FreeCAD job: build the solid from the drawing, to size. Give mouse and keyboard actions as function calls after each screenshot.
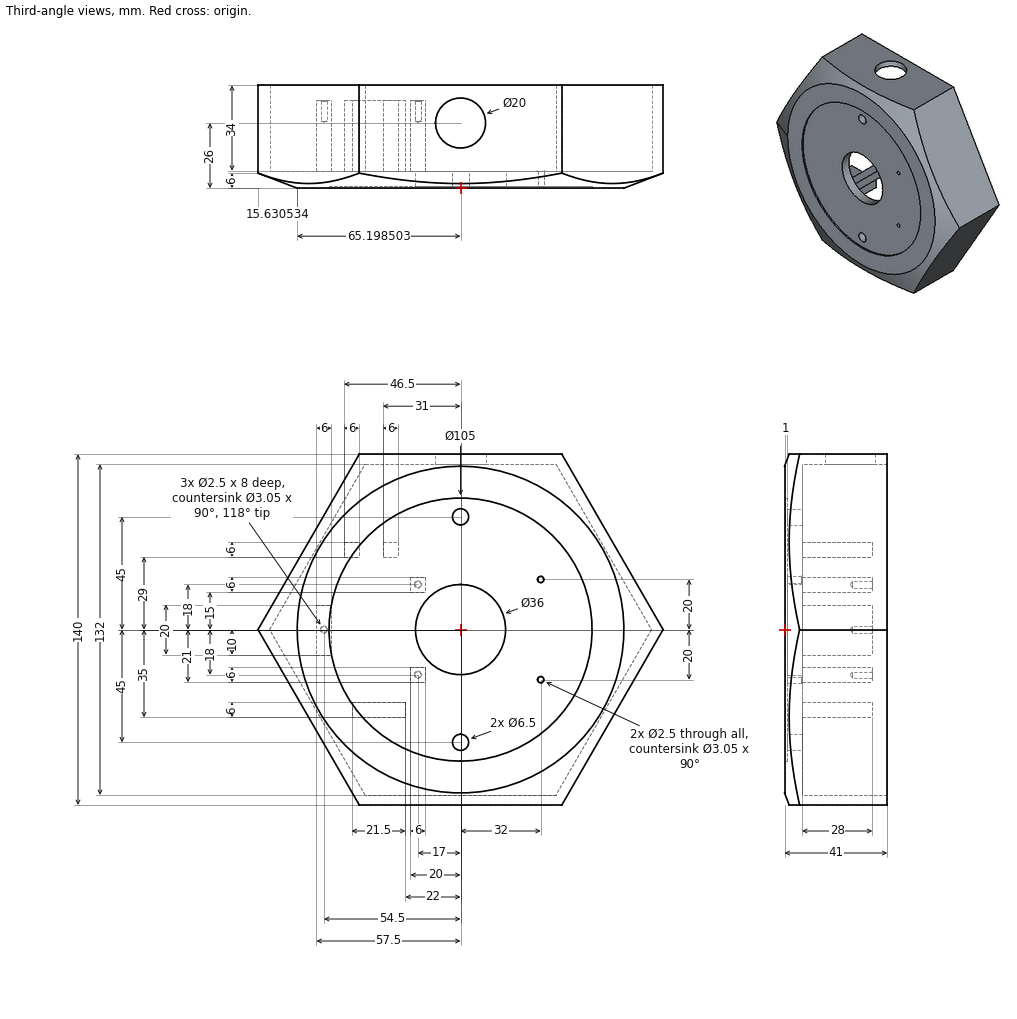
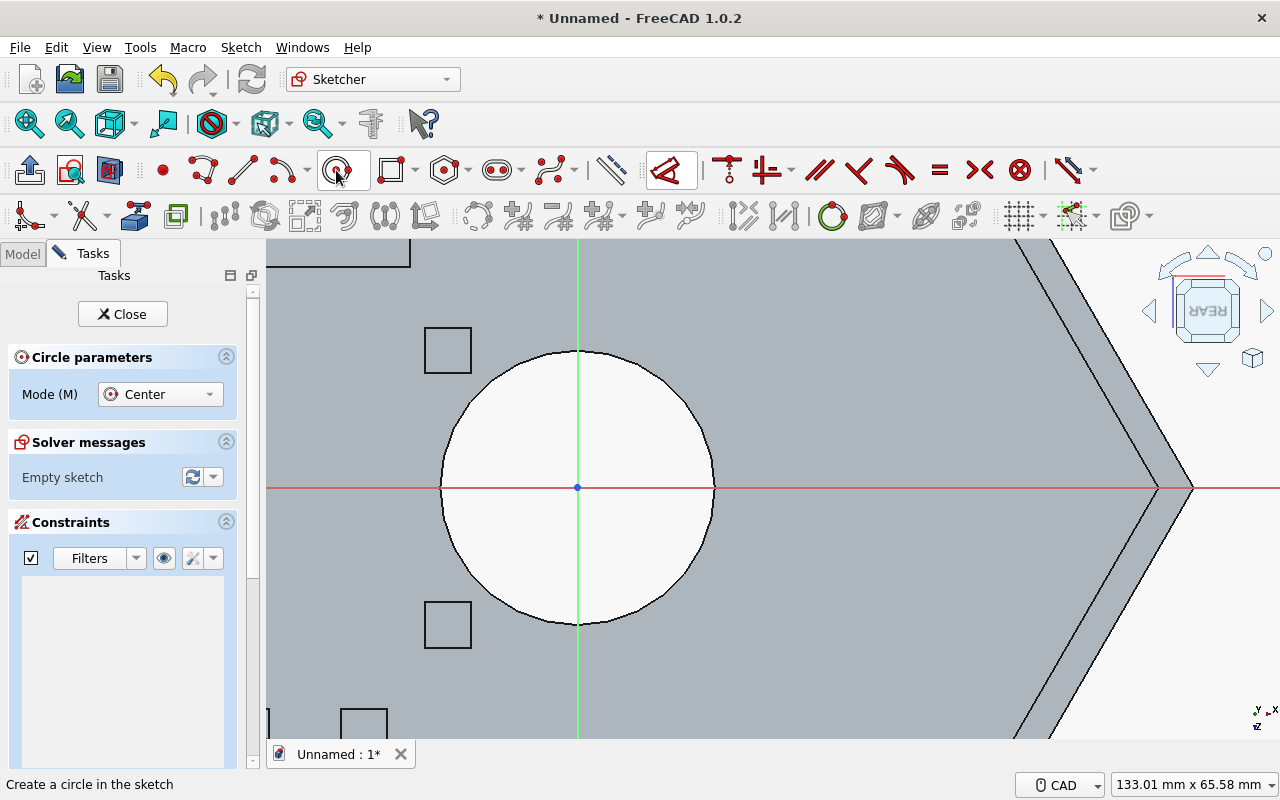
scroll(821, 335, up, 5)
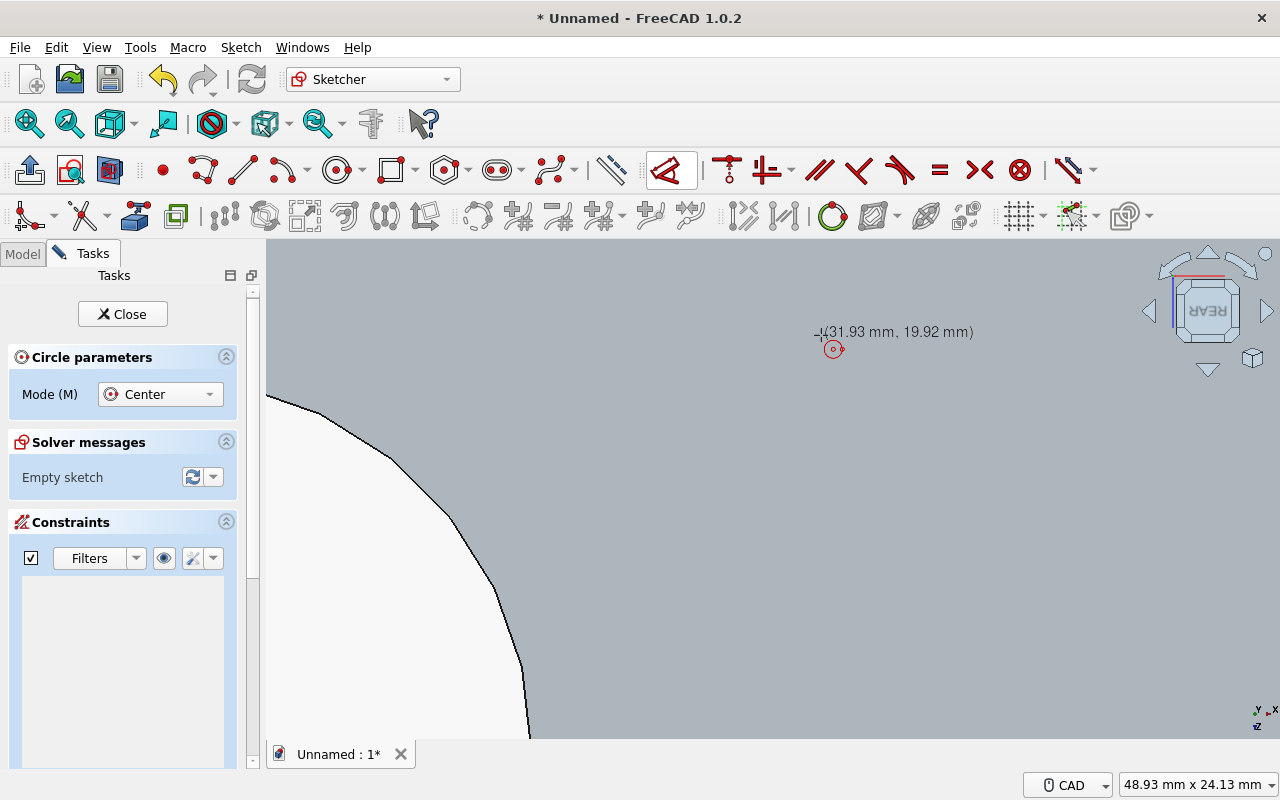
click(821, 336)
move(840, 317)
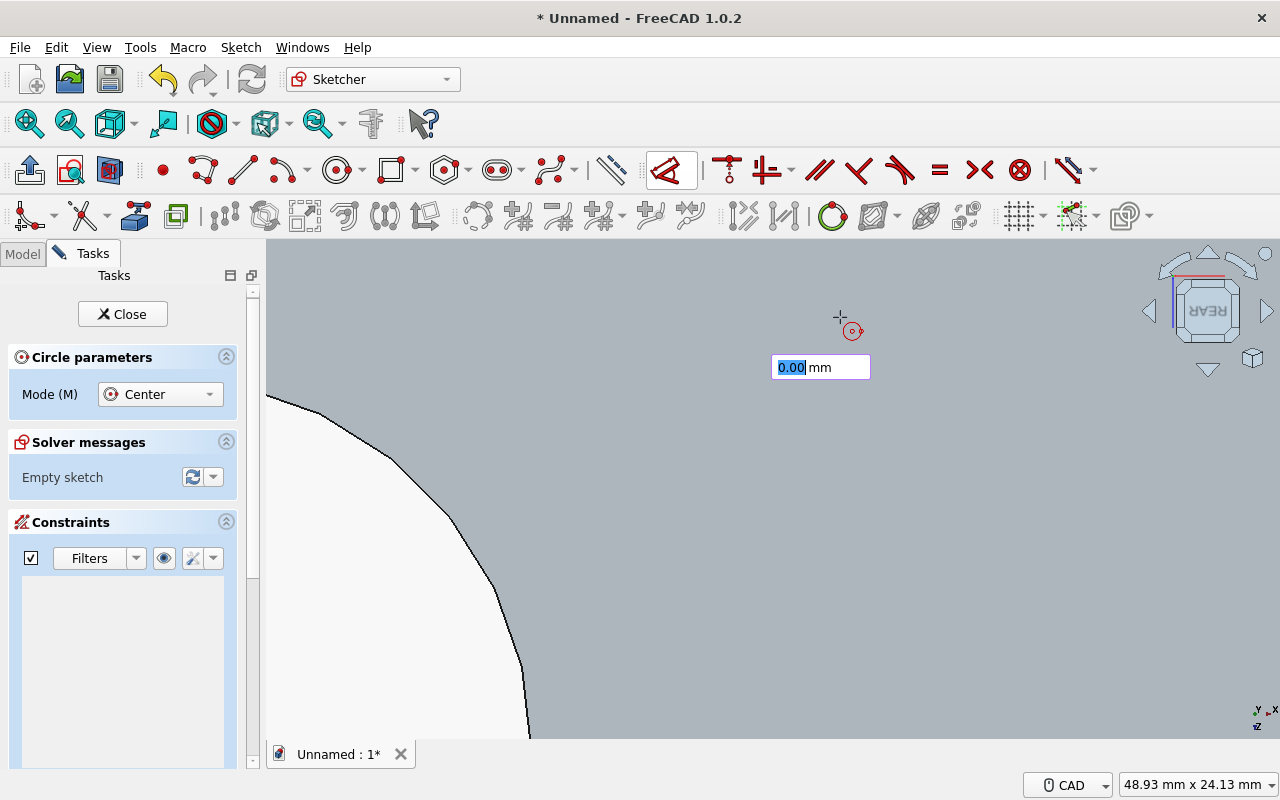
text(2.5)
key(Return)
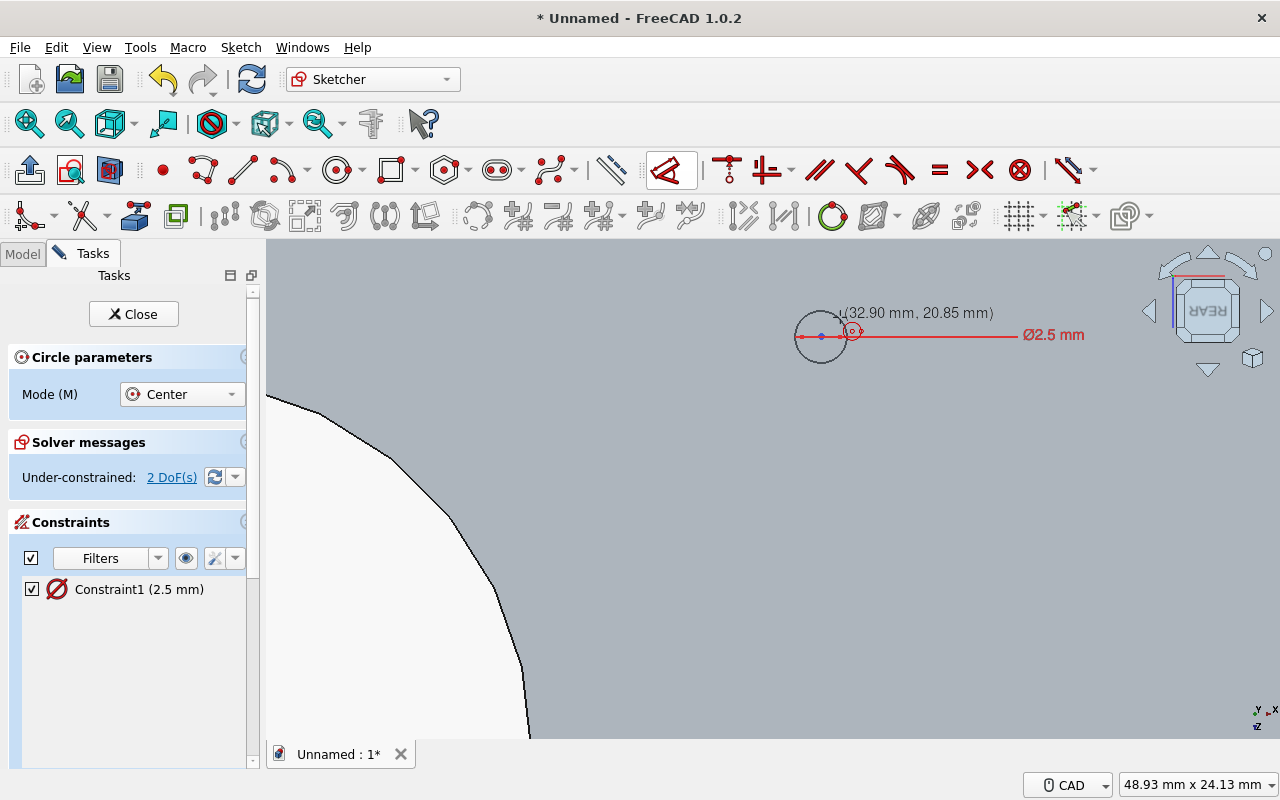
scroll(822, 337, down, 5)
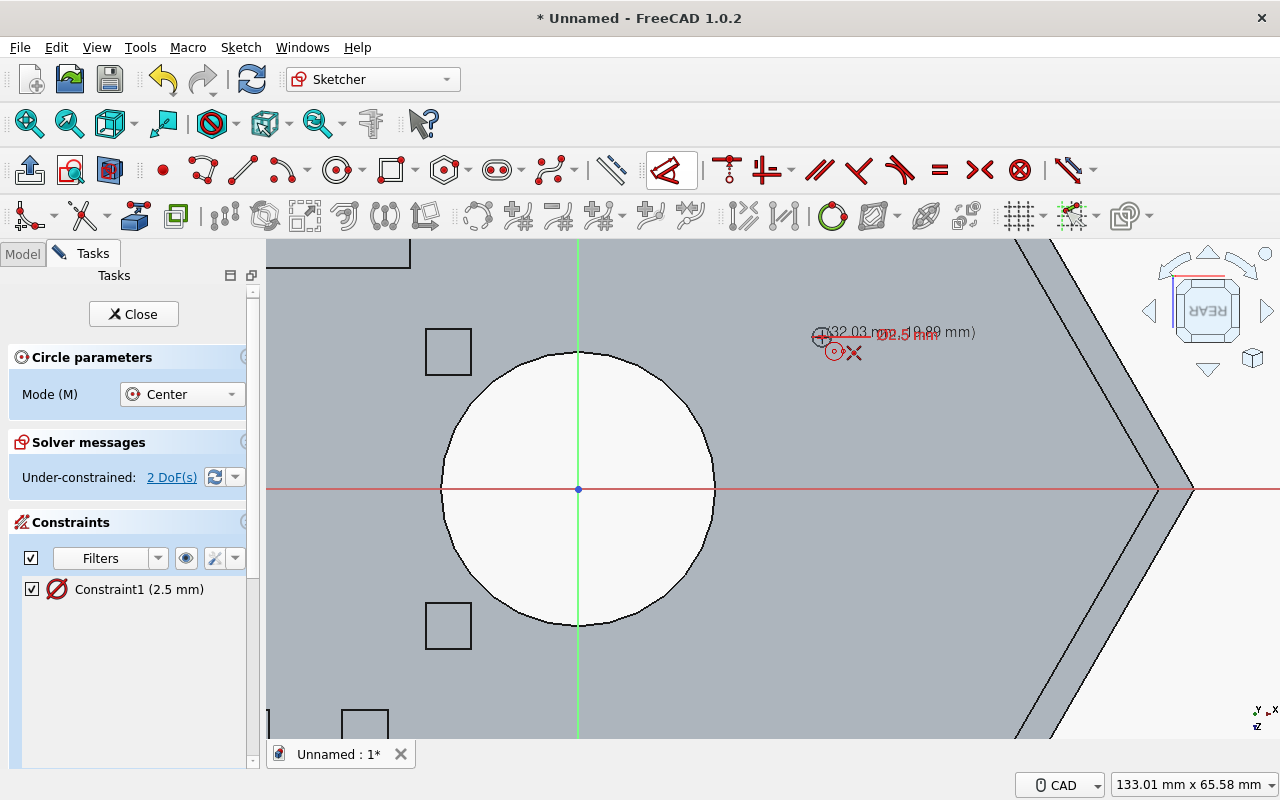
scroll(822, 642, up, 5)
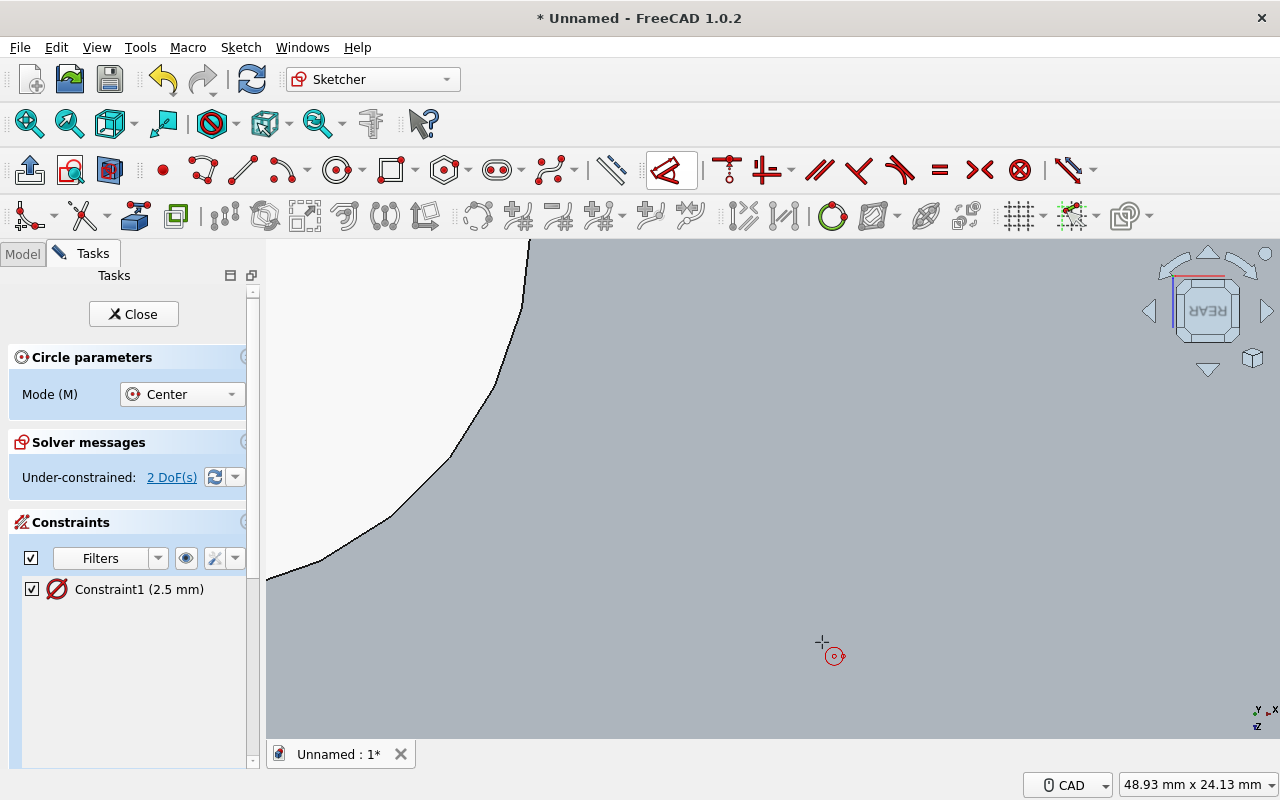
click(821, 639)
move(840, 621)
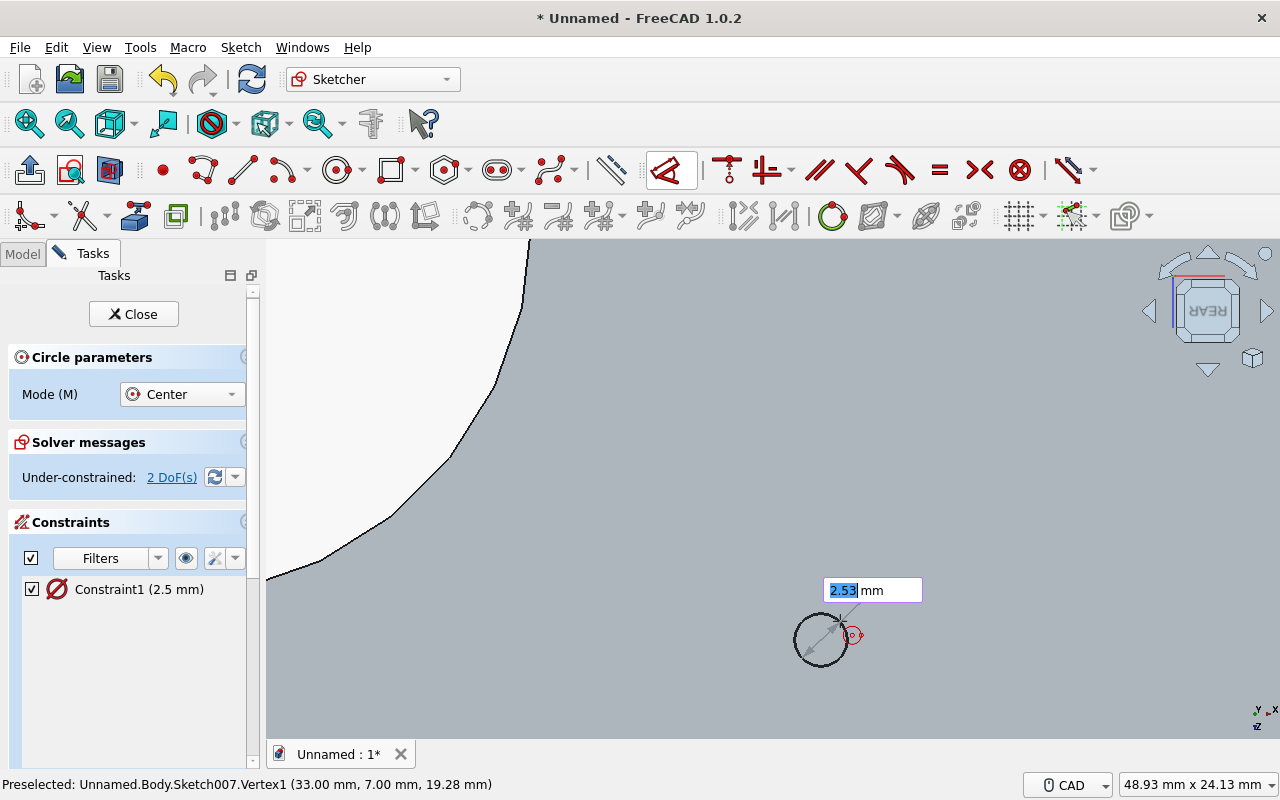
text(2.5)
key(Return)
key(Escape)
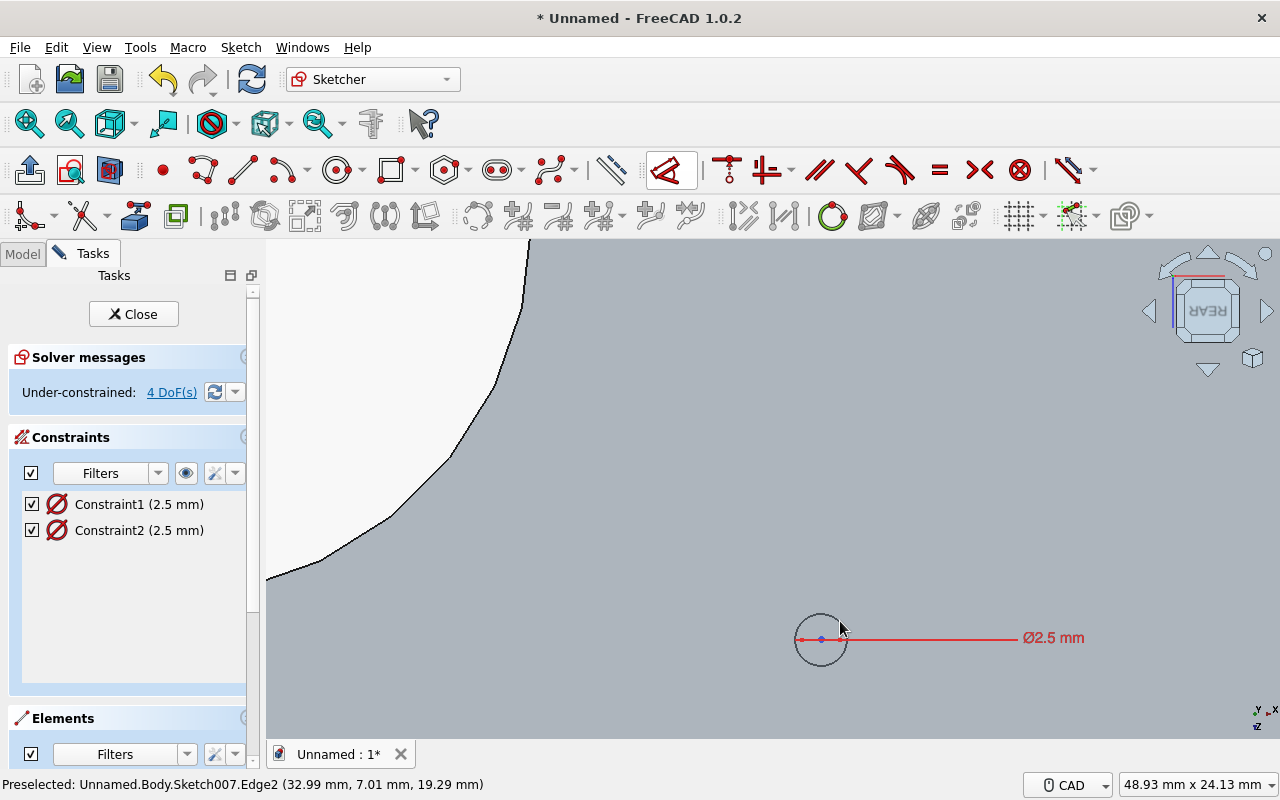
scroll(822, 643, down, 5)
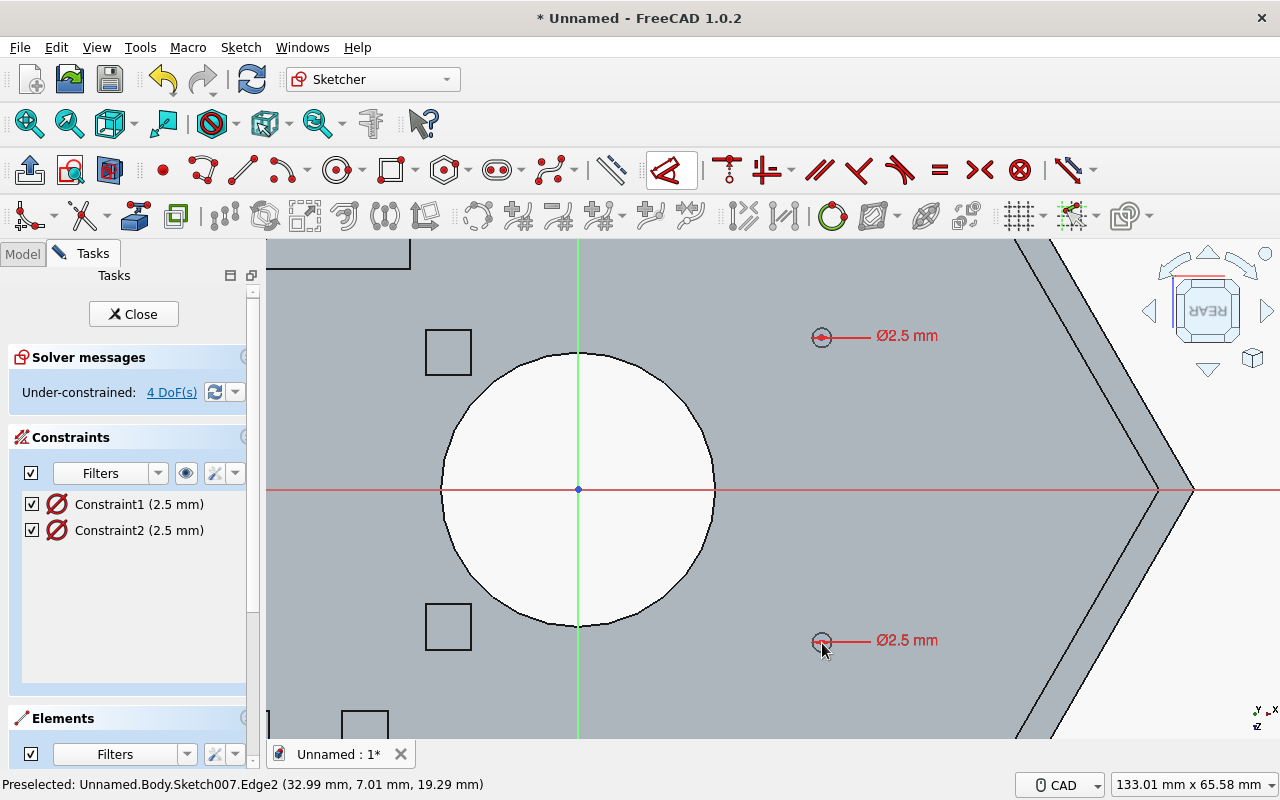
click(822, 338)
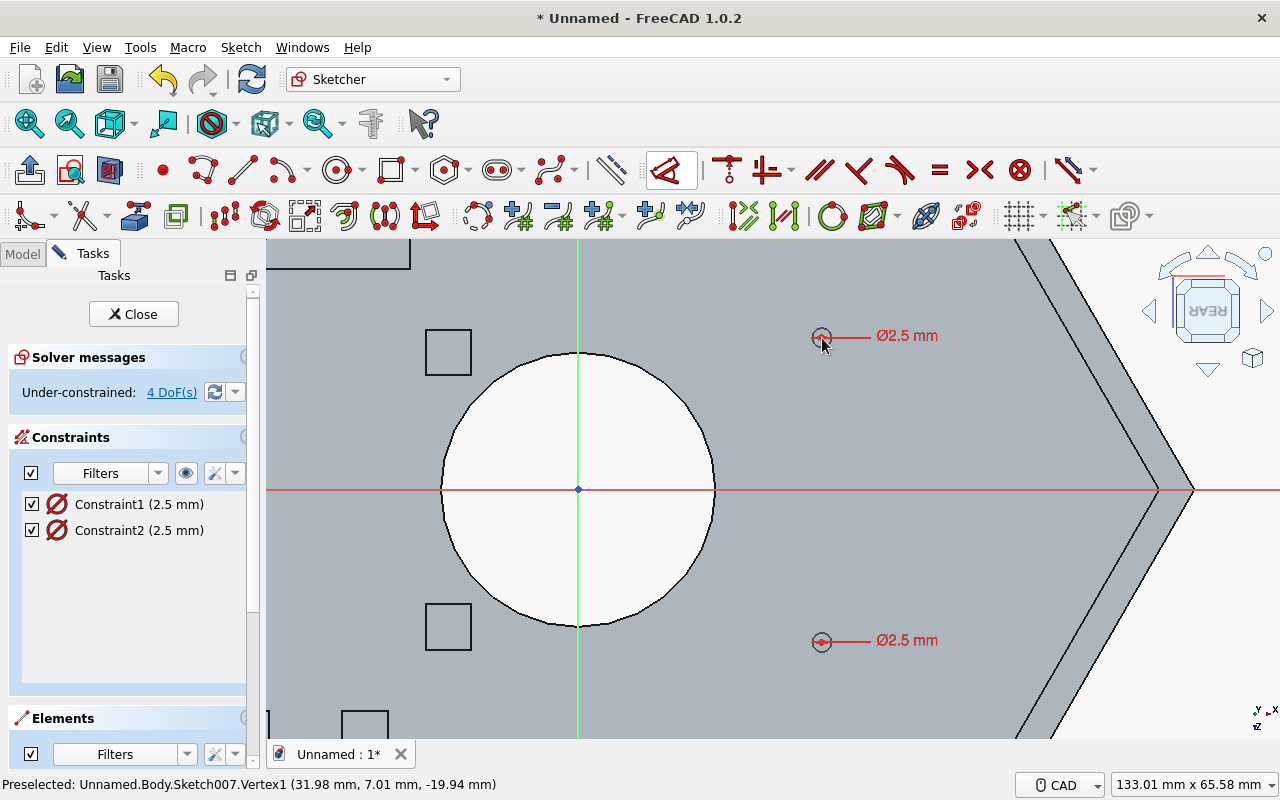
click(822, 642)